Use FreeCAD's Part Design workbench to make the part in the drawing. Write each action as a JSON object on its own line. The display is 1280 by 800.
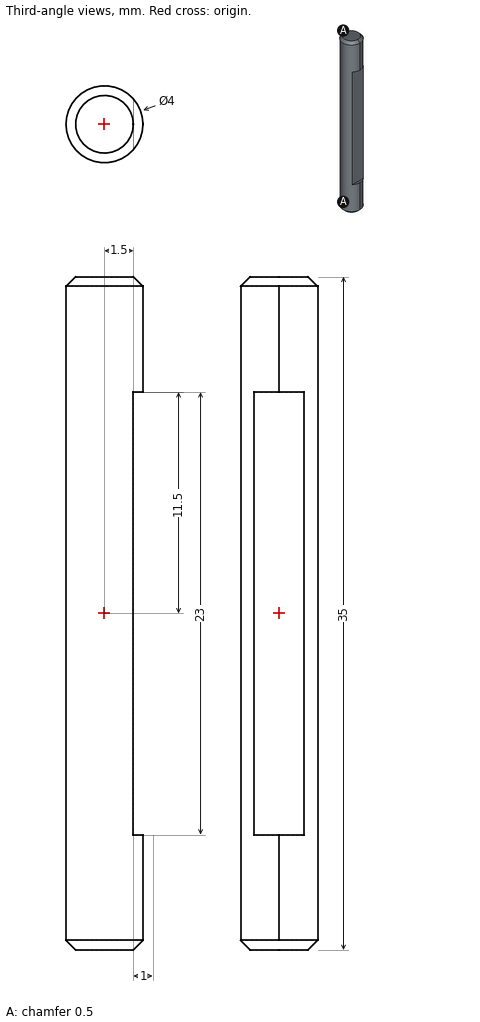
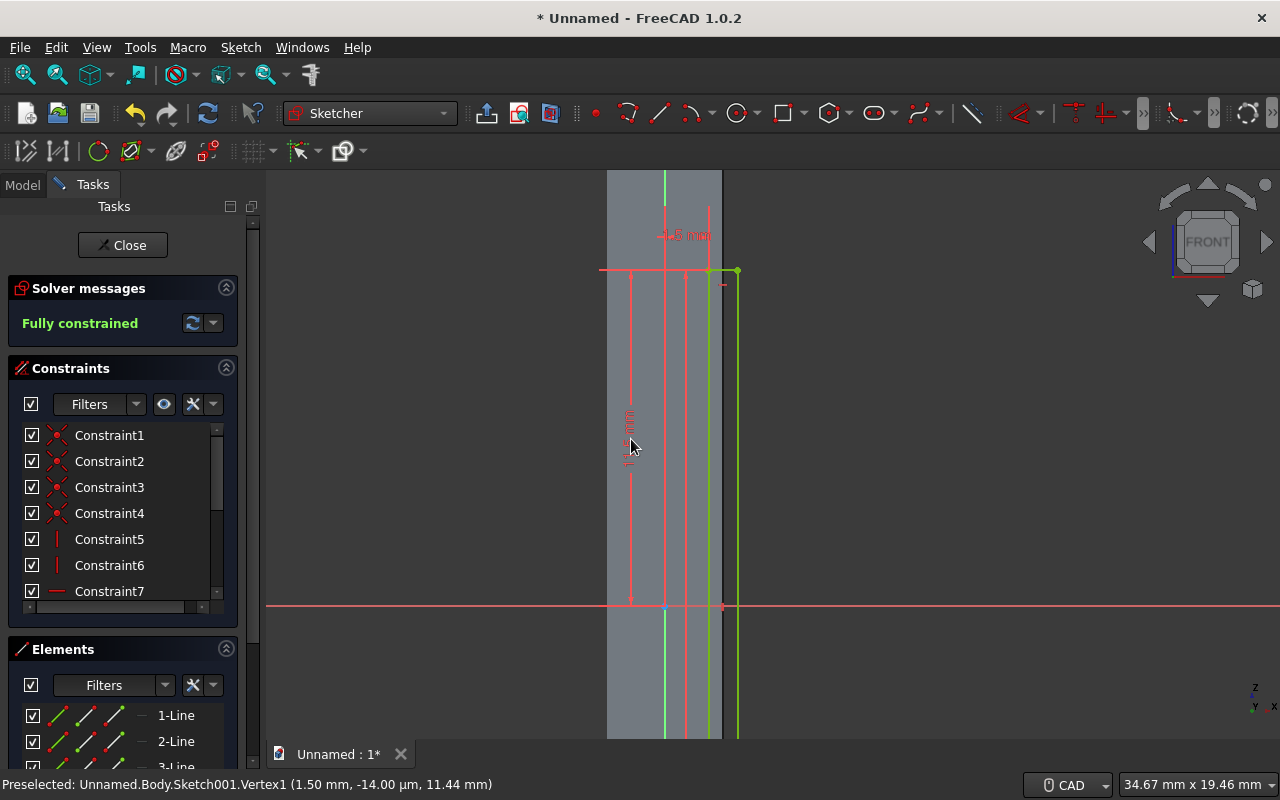
{"action": "left_click", "coordinate": [123, 245]}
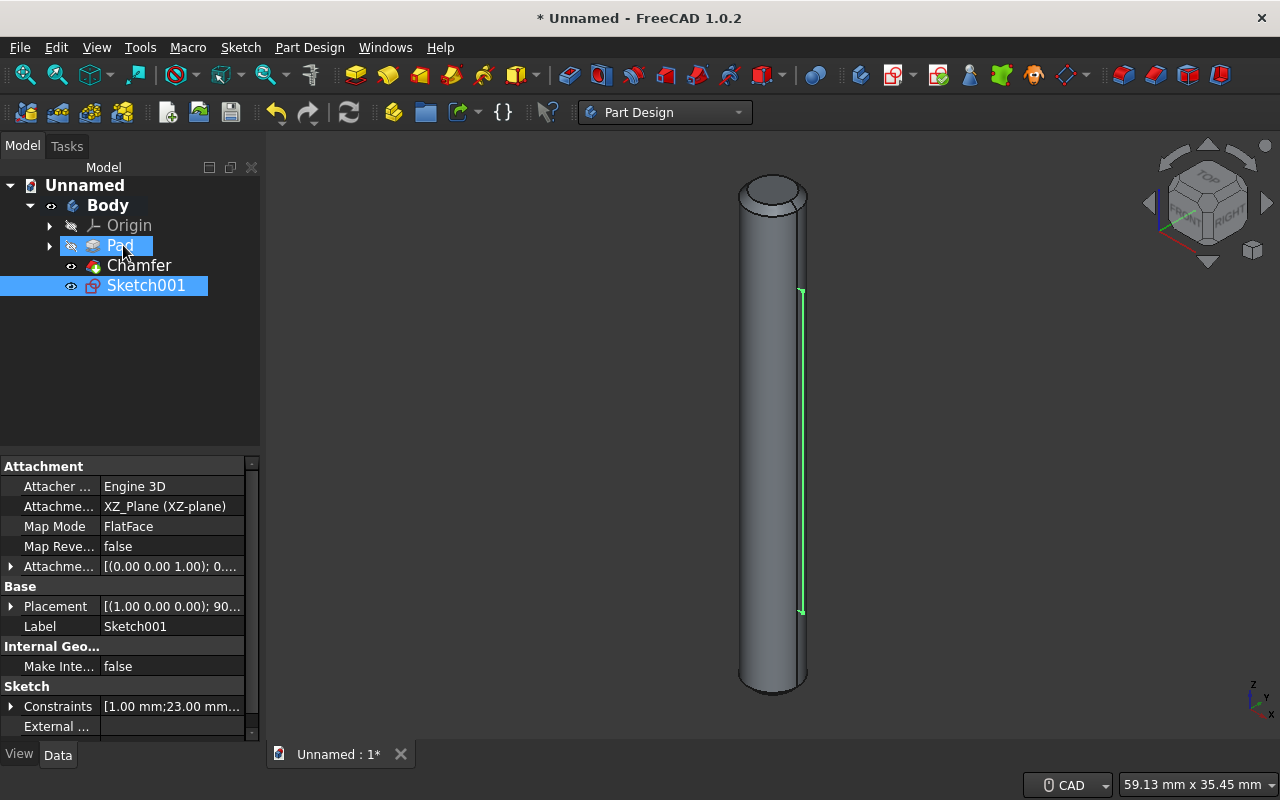
{"action": "left_click", "coordinate": [570, 76]}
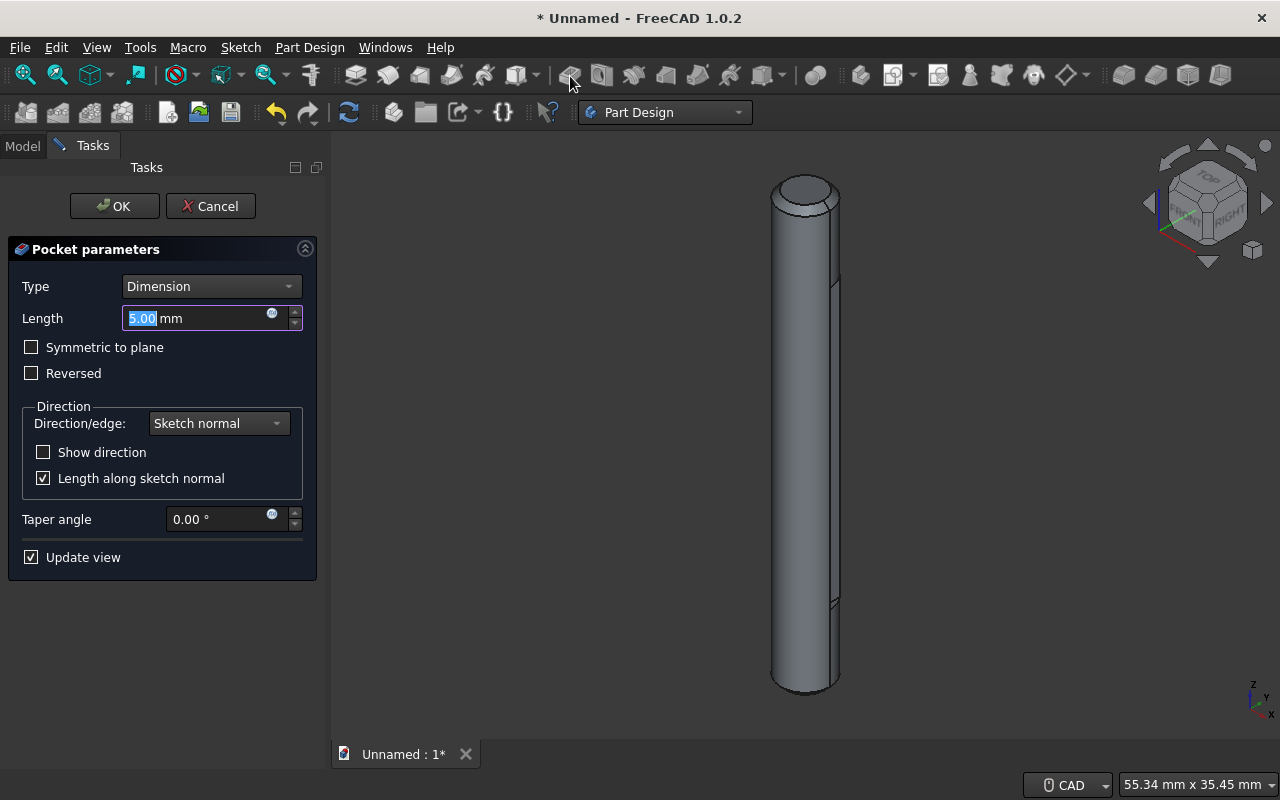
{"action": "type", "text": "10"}
{"action": "key", "text": "Tab"}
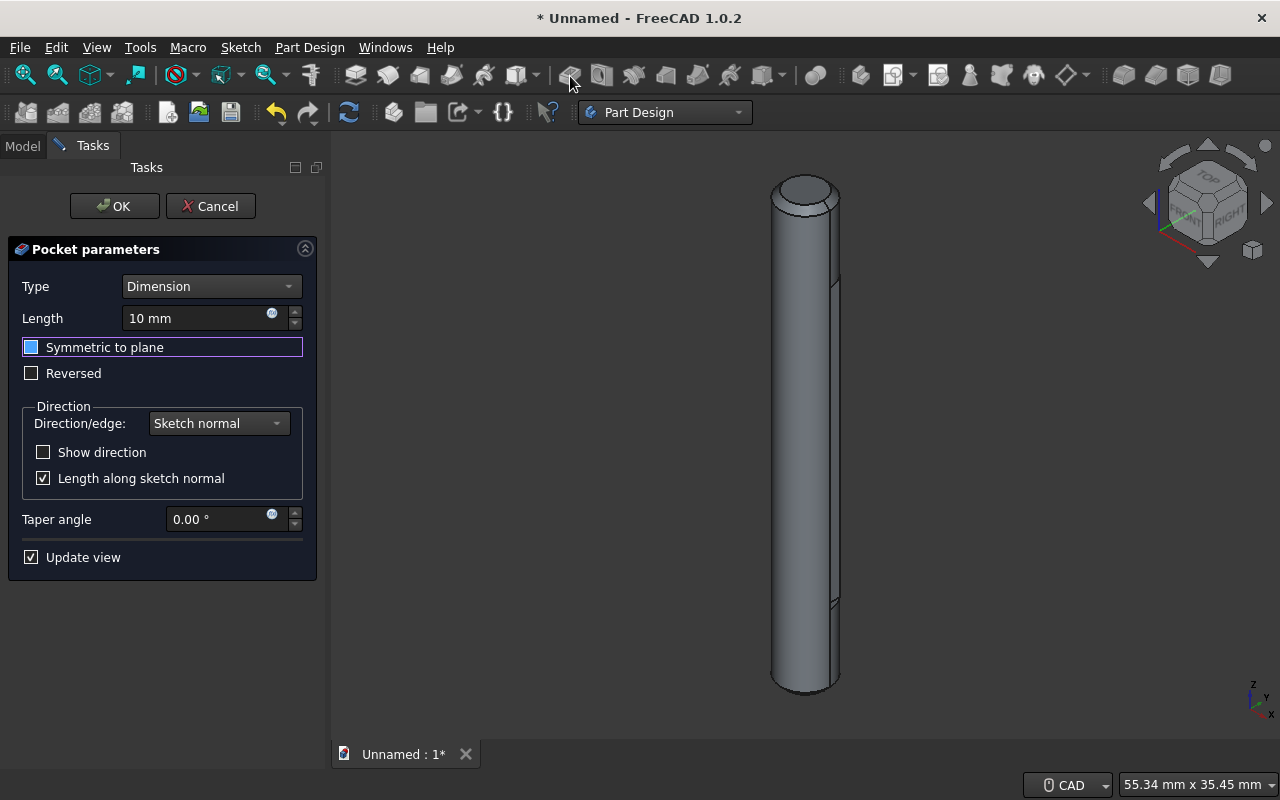
{"action": "left_click", "coordinate": [30, 347]}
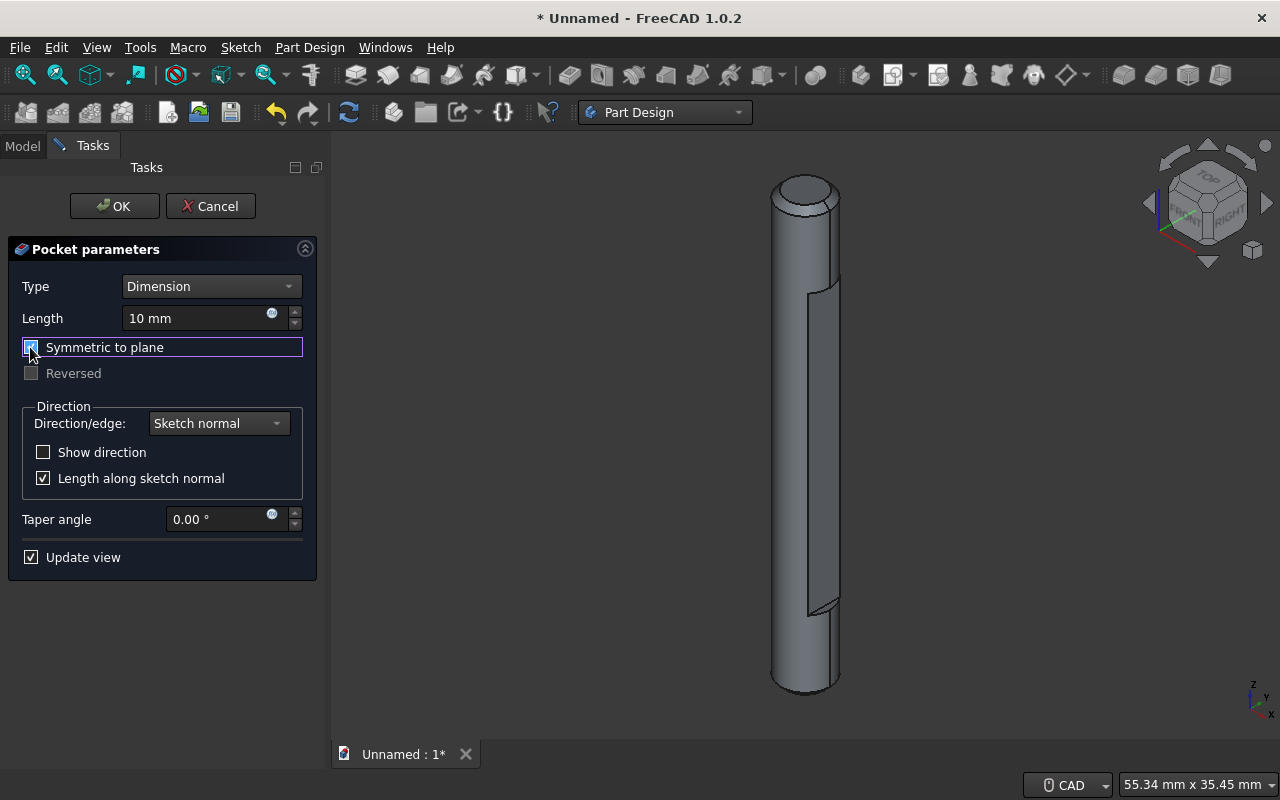
{"action": "left_click", "coordinate": [115, 206]}